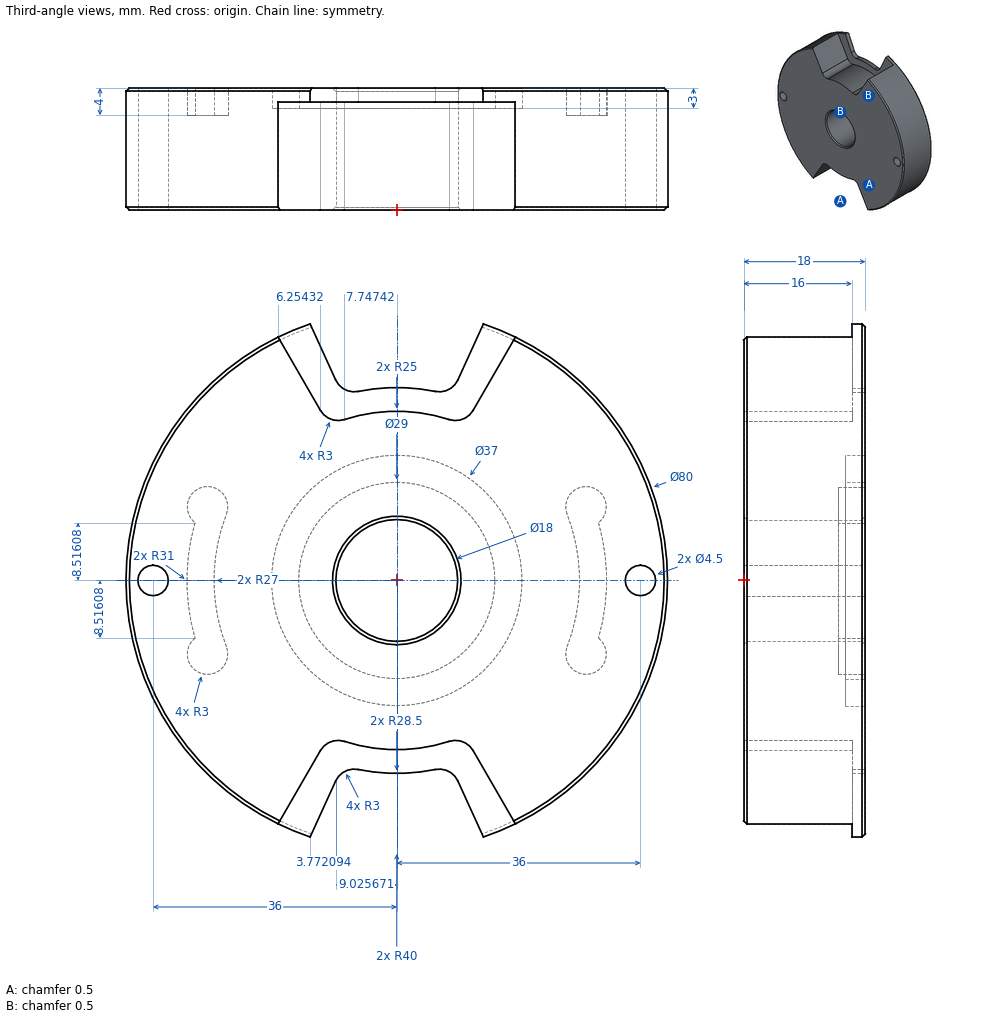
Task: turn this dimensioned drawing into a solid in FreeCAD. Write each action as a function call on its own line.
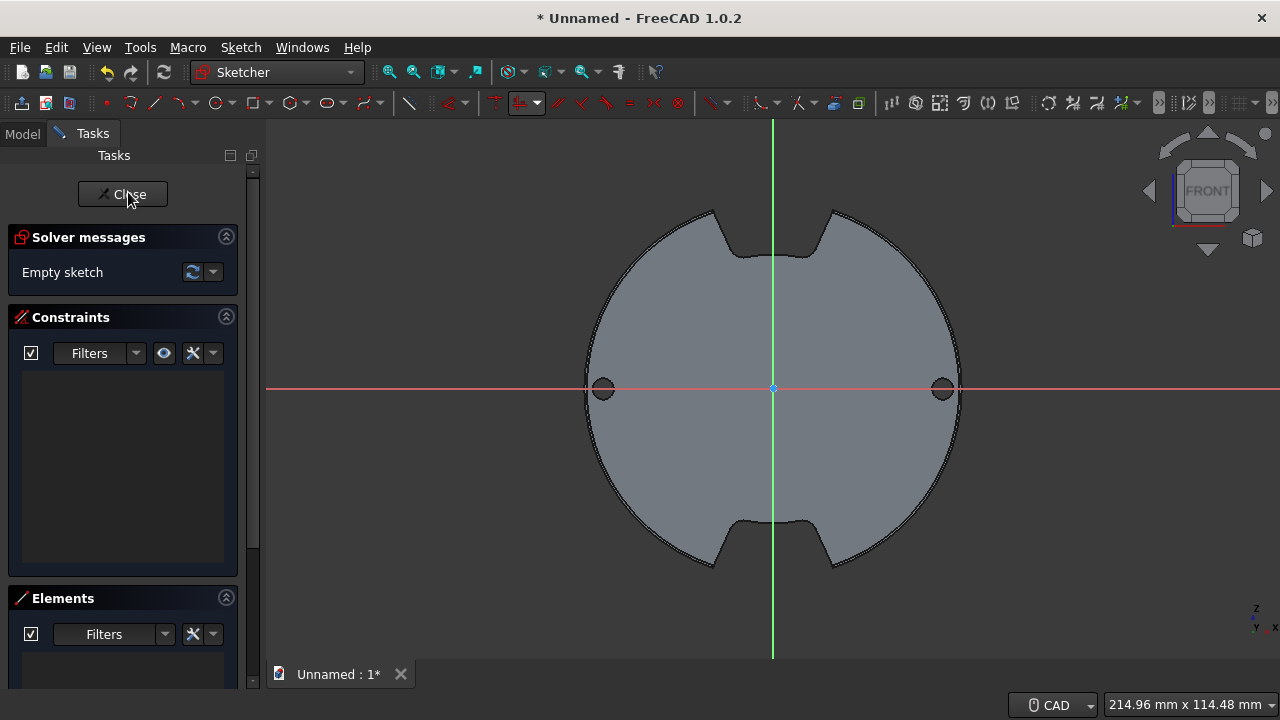
scroll(795, 389, up, 7)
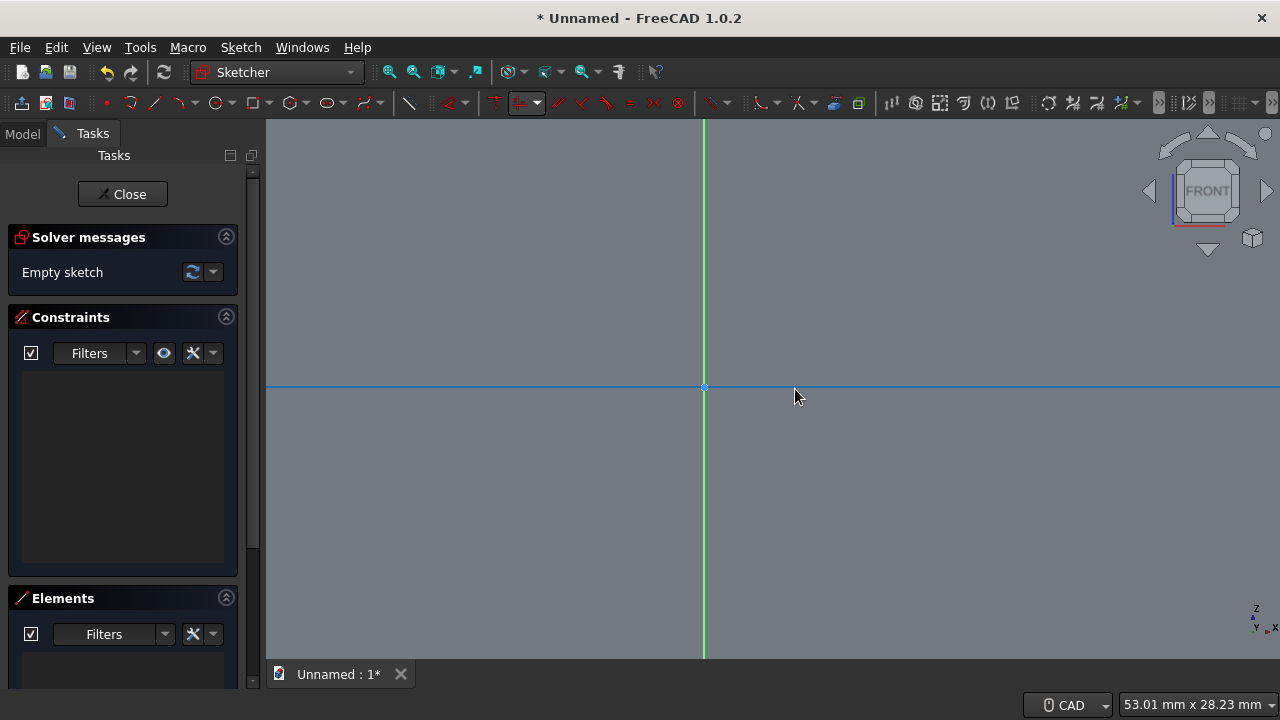
click(216, 104)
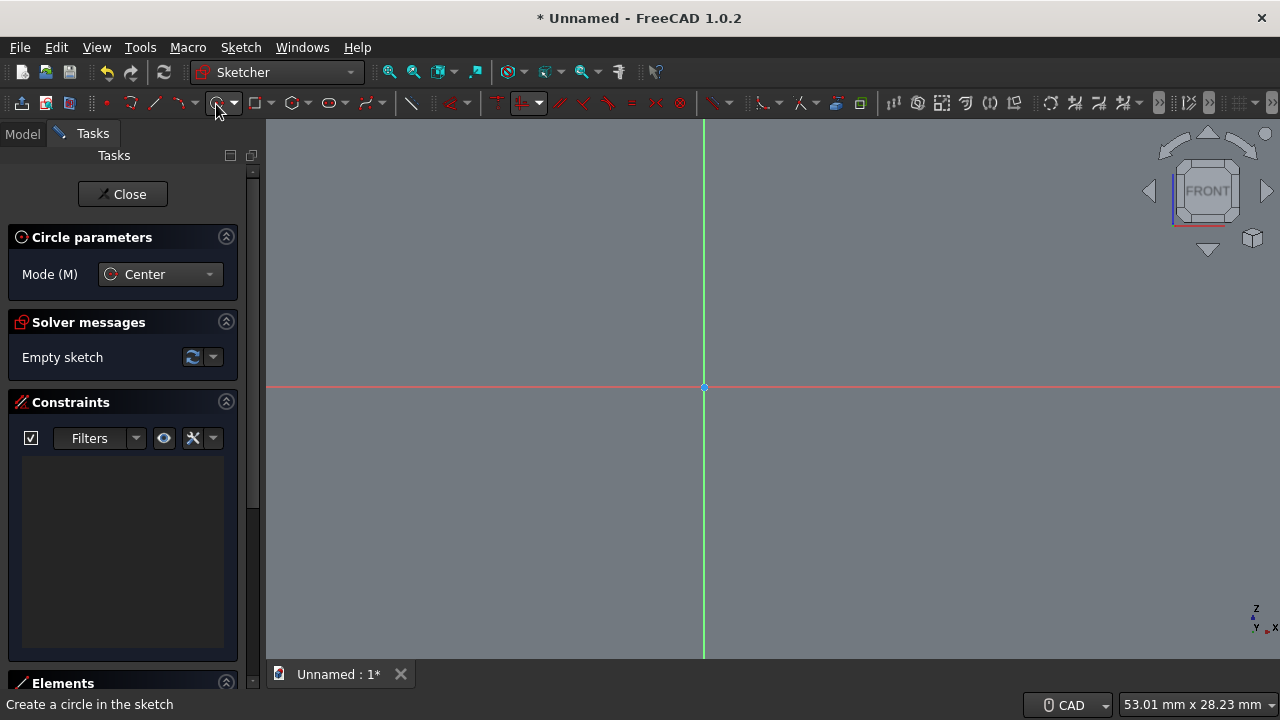
click(704, 387)
click(826, 266)
key(Escape)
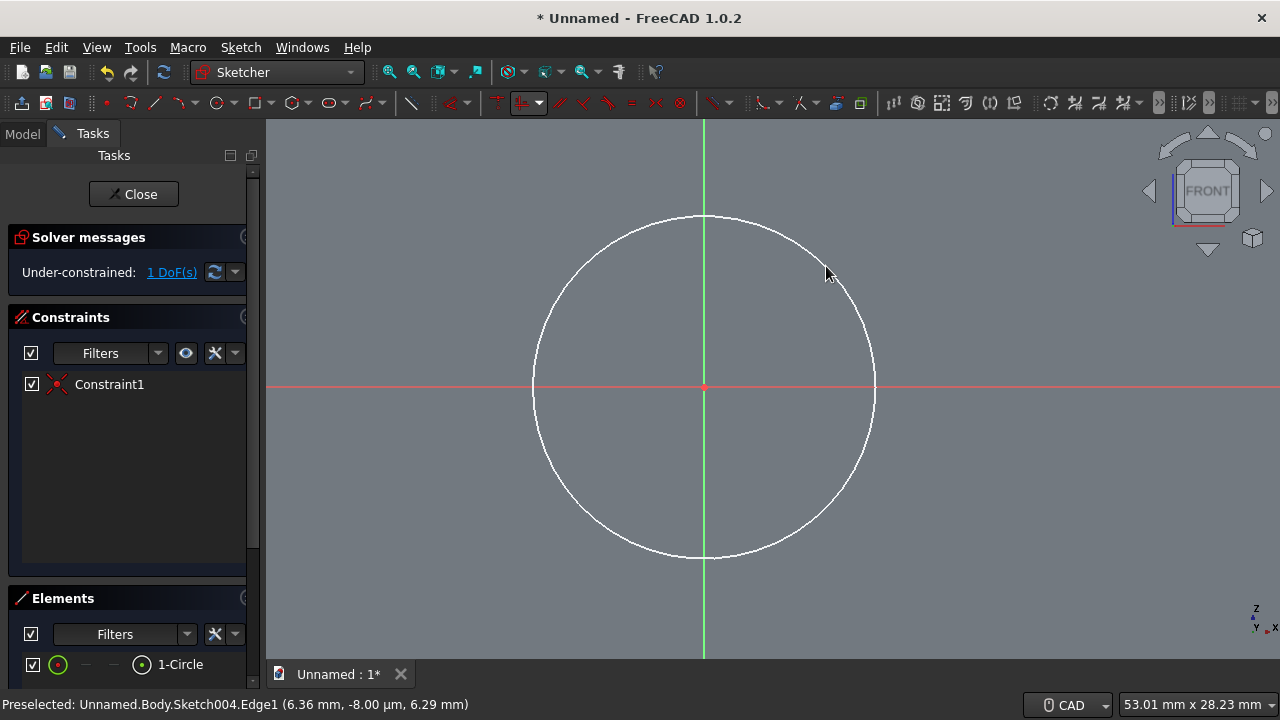
click(450, 104)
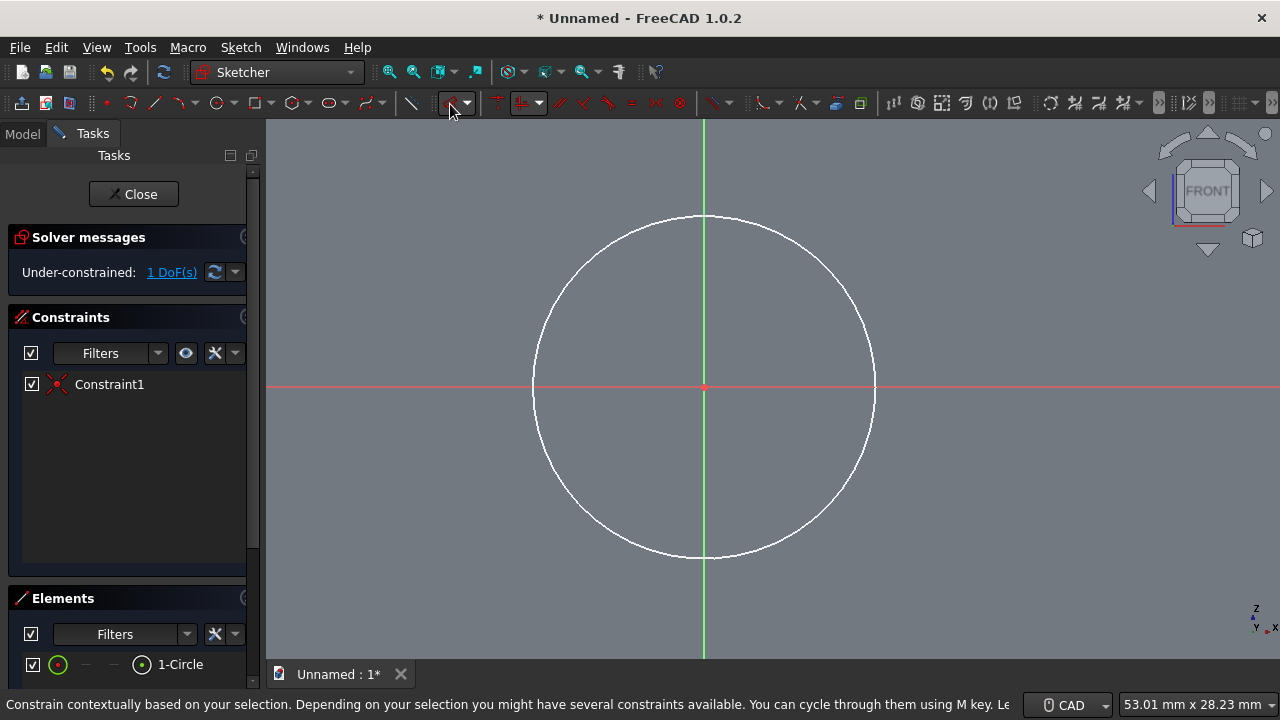
click(825, 266)
click(848, 243)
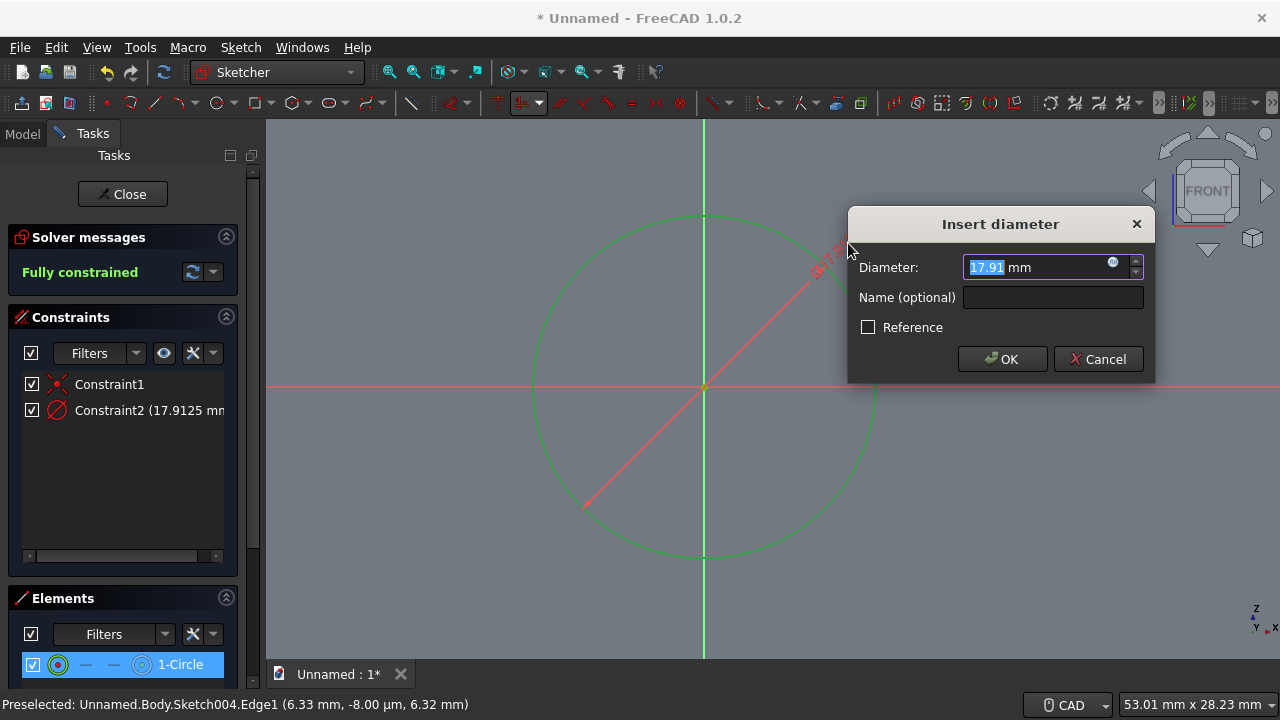
text(18)
key(Return)
key(Escape)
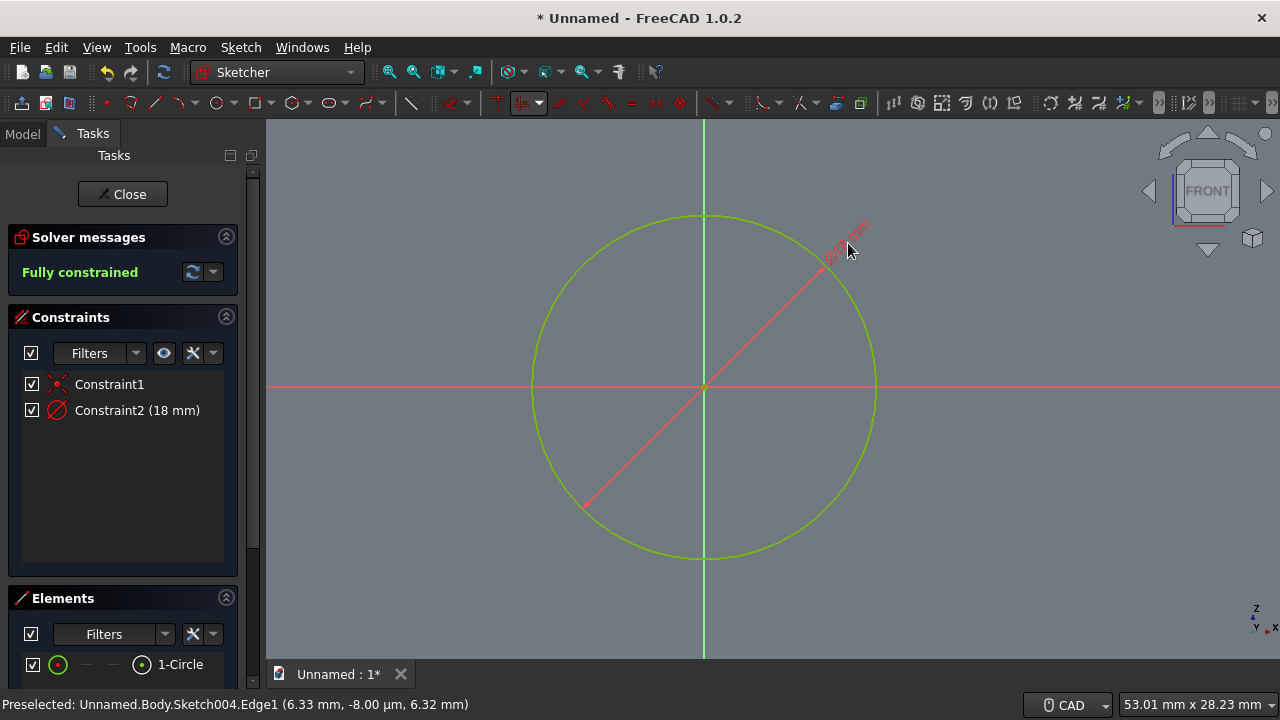
click(123, 194)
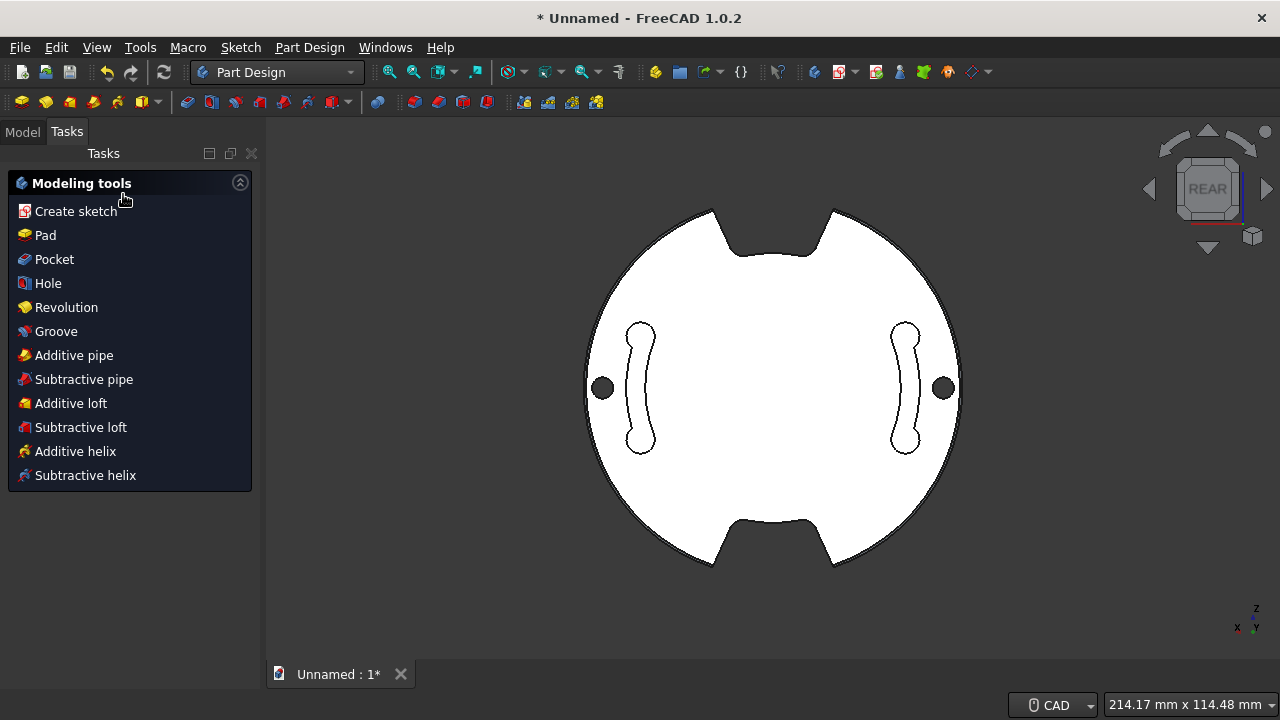
click(188, 102)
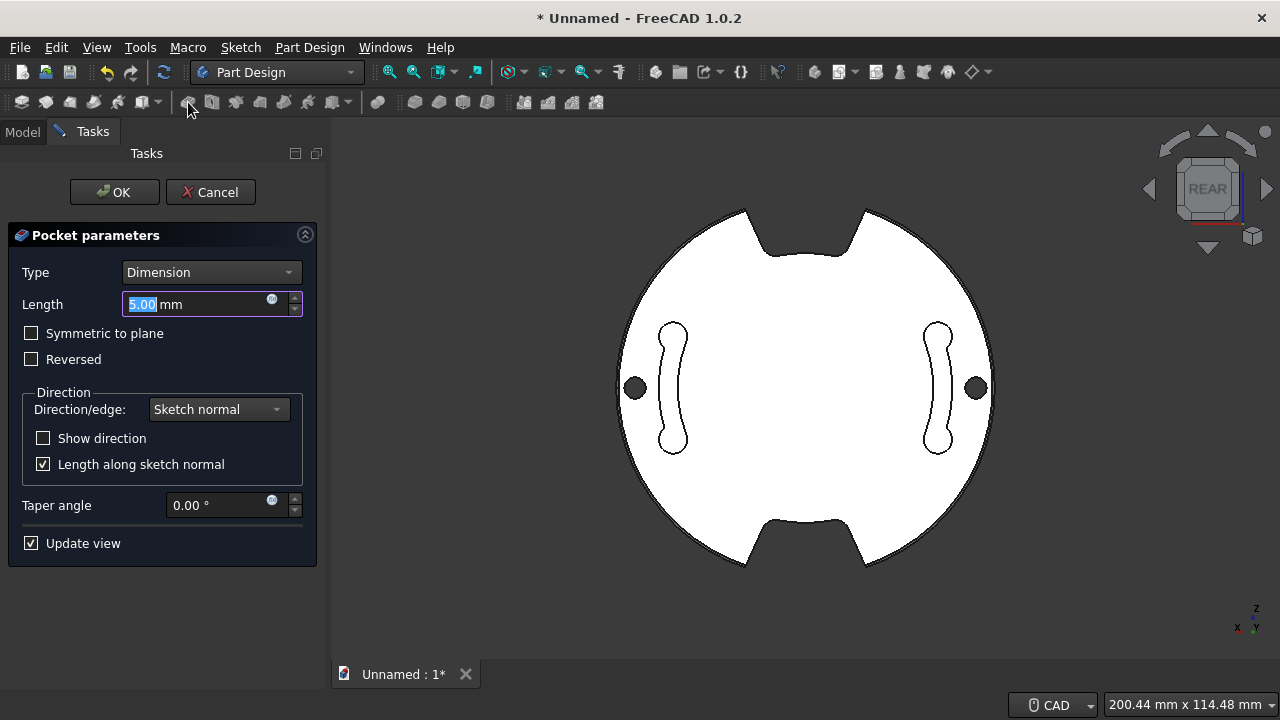
click(212, 272)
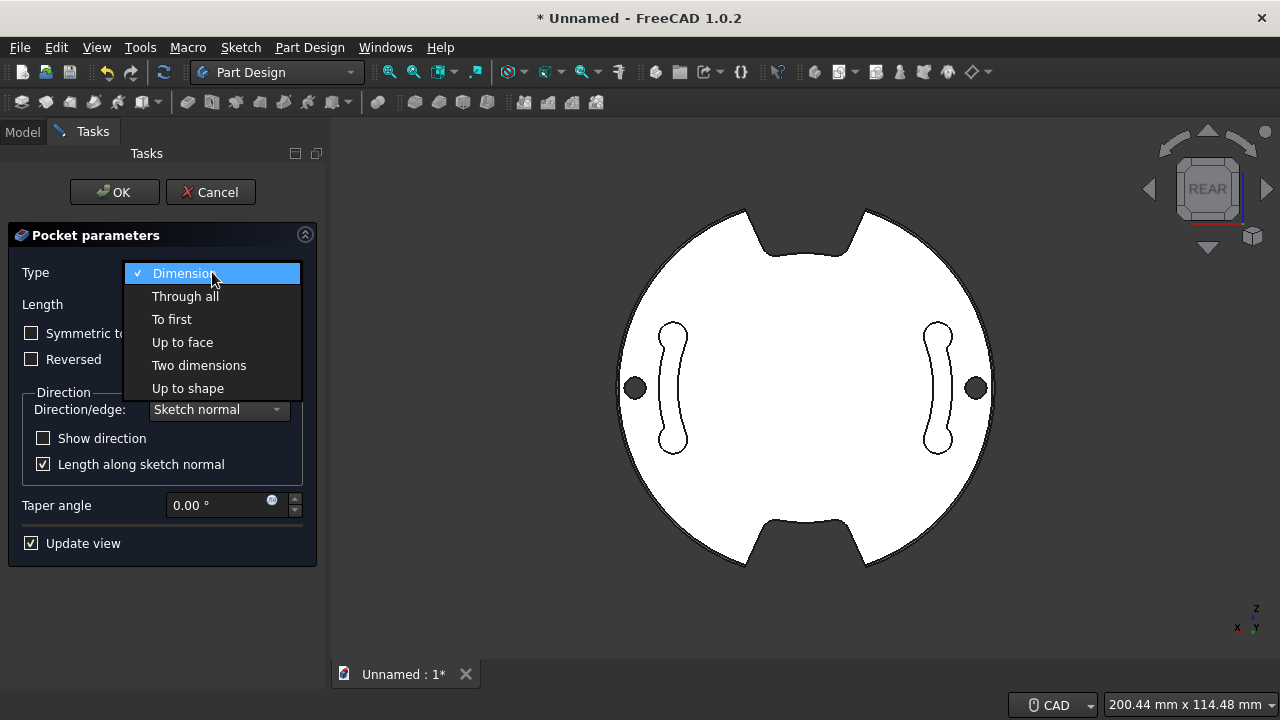
click(212, 296)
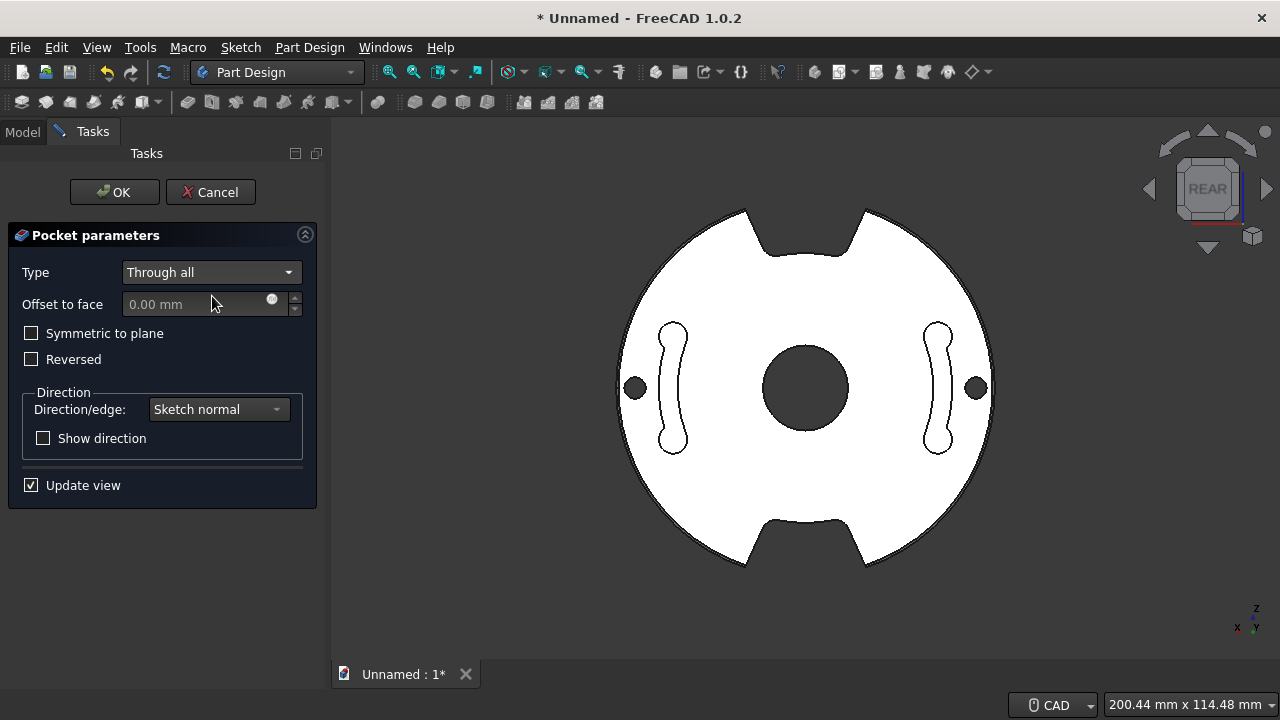
click(115, 192)